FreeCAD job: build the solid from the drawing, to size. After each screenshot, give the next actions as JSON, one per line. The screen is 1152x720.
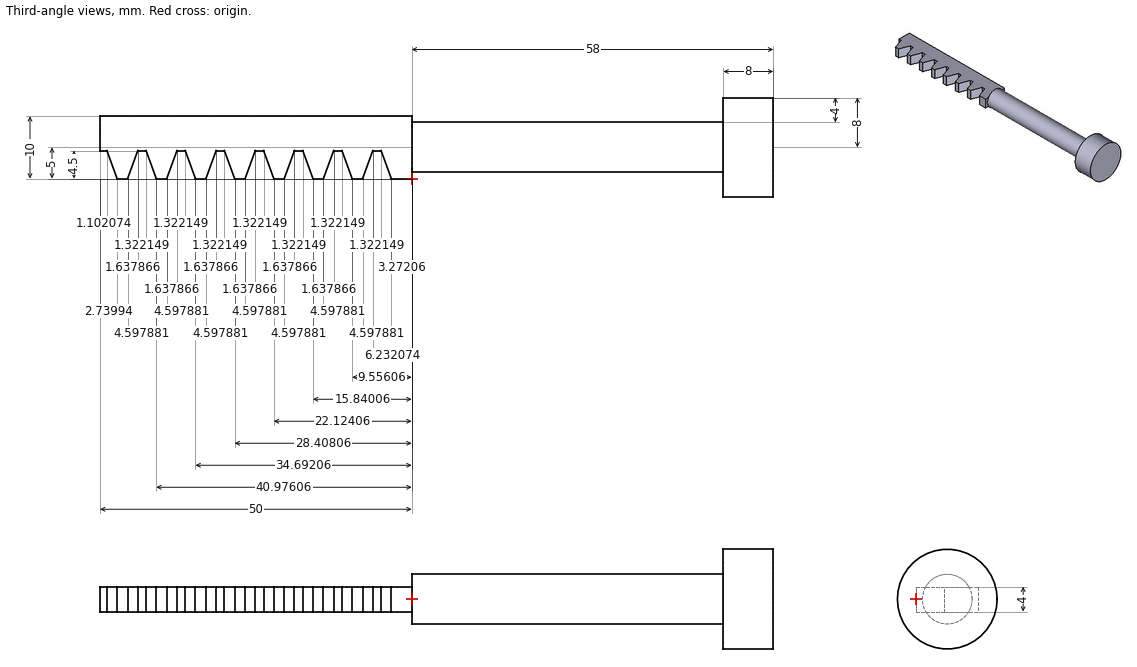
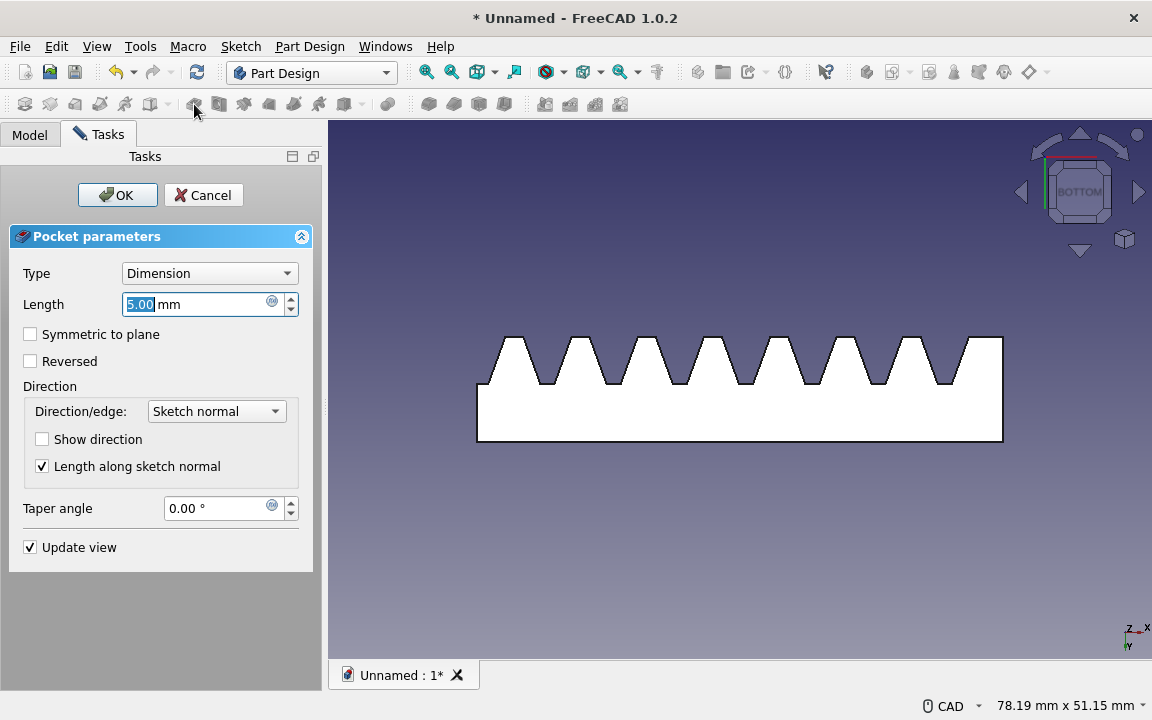
{"action": "left_click", "coordinate": [210, 274]}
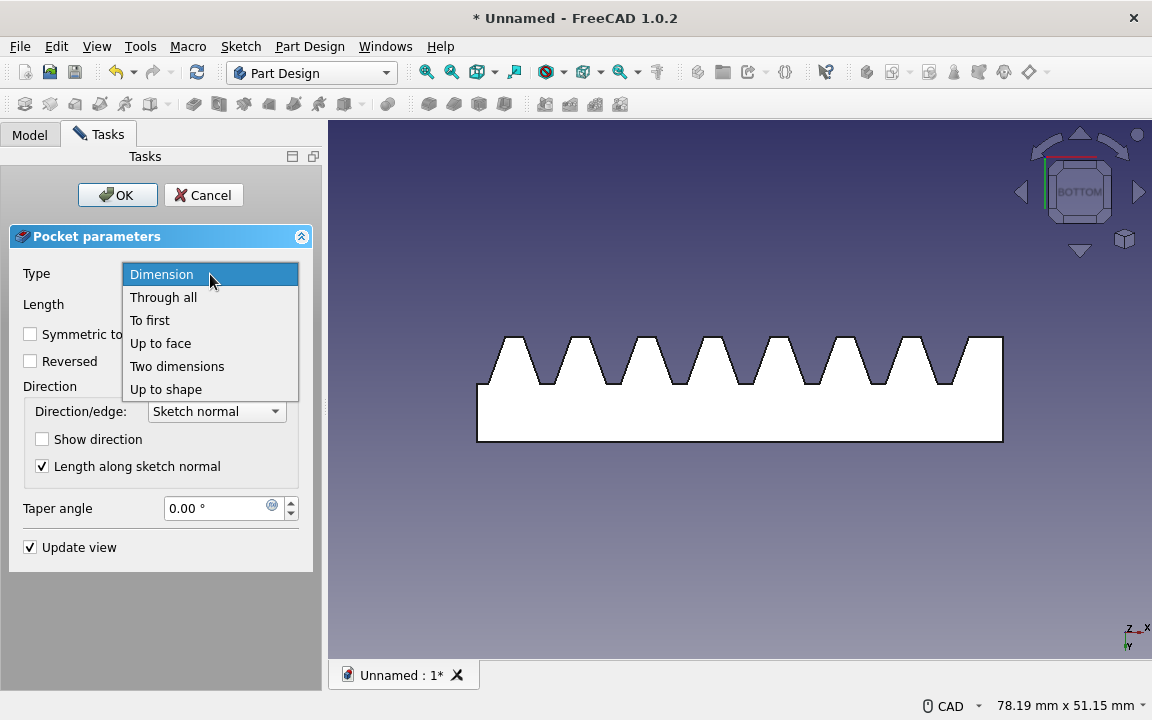
{"action": "left_click", "coordinate": [208, 298]}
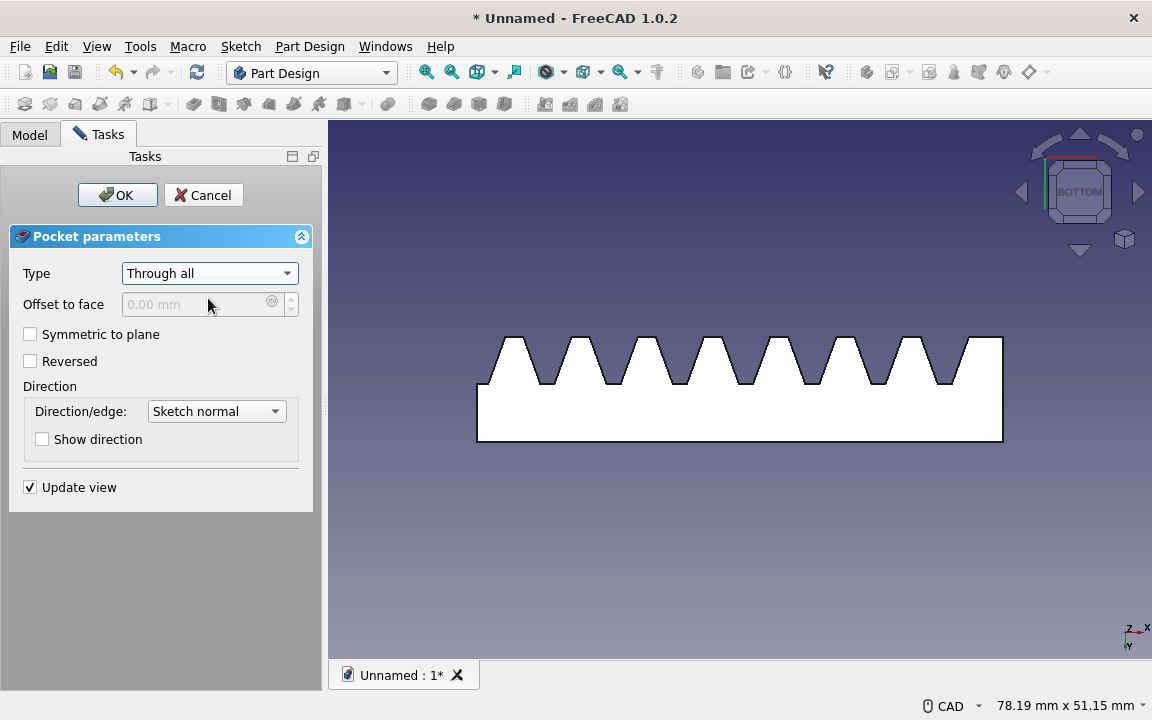
{"action": "left_click", "coordinate": [118, 195]}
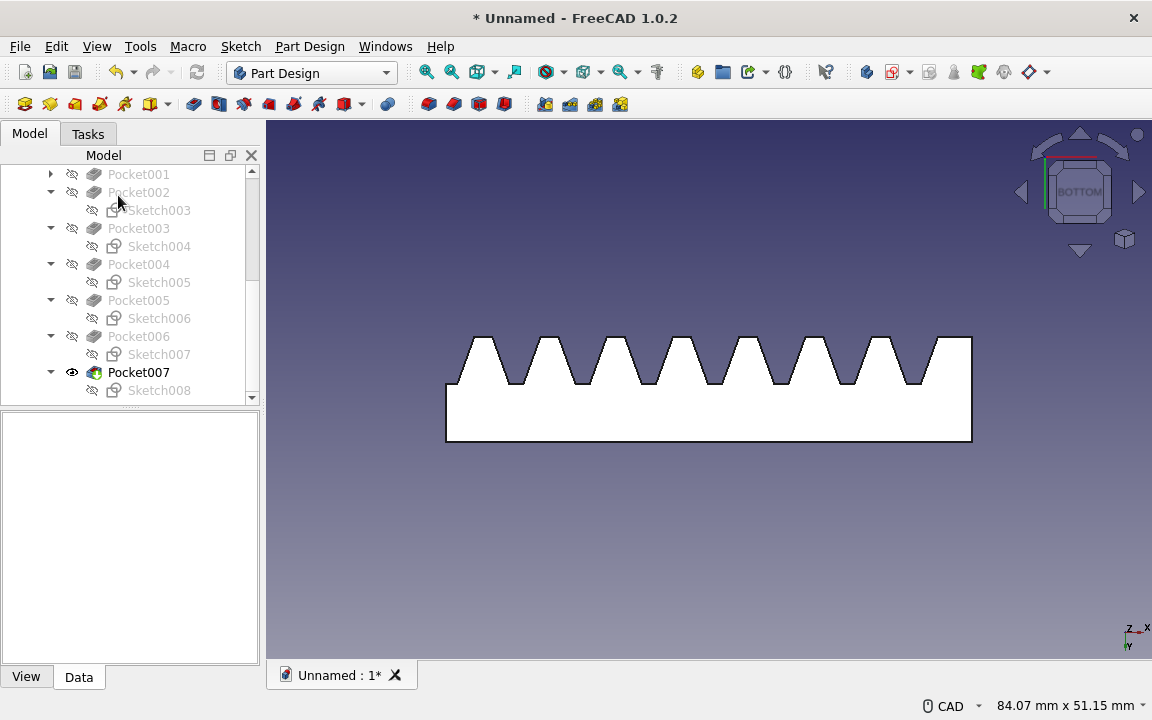
{"action": "left_click", "coordinate": [892, 72]}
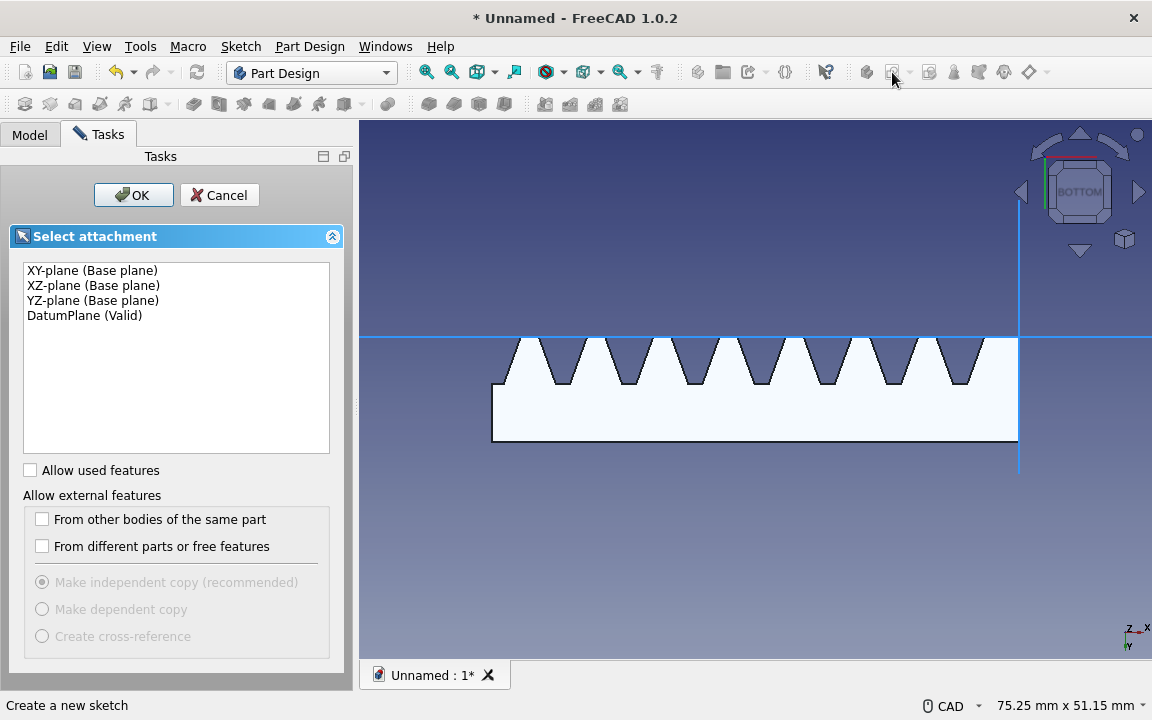
{"action": "left_click", "coordinate": [84, 270]}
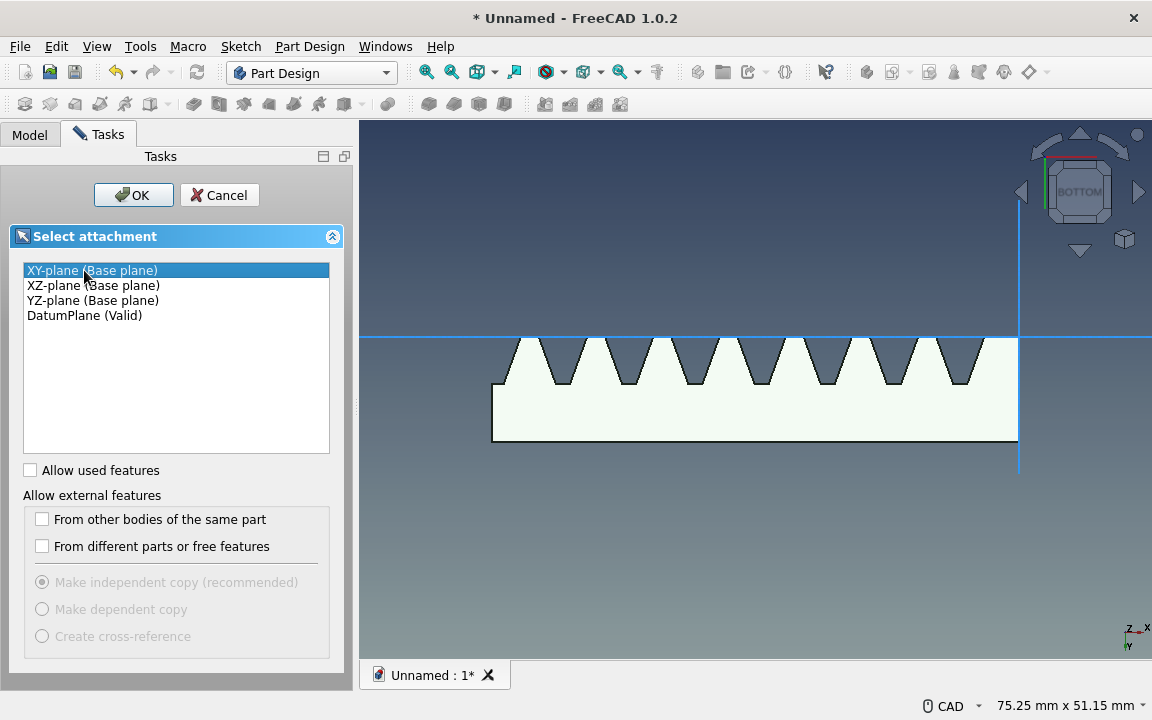
{"action": "left_click", "coordinate": [134, 195]}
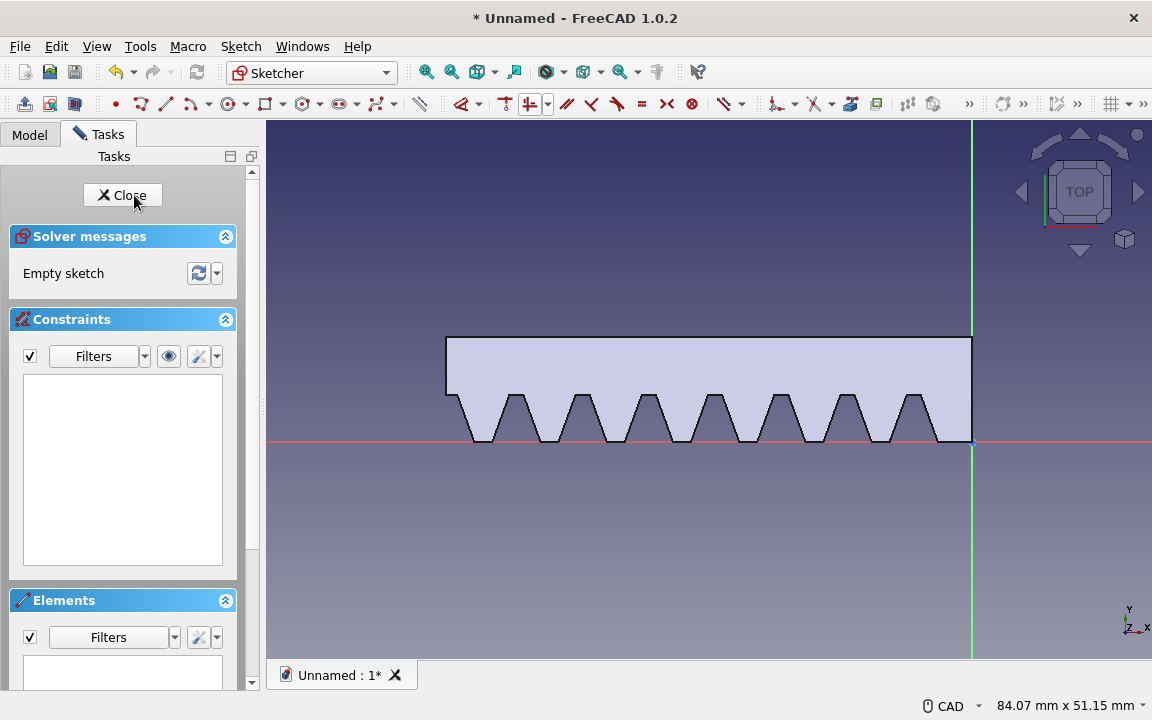
{"action": "left_click", "coordinate": [75, 104]}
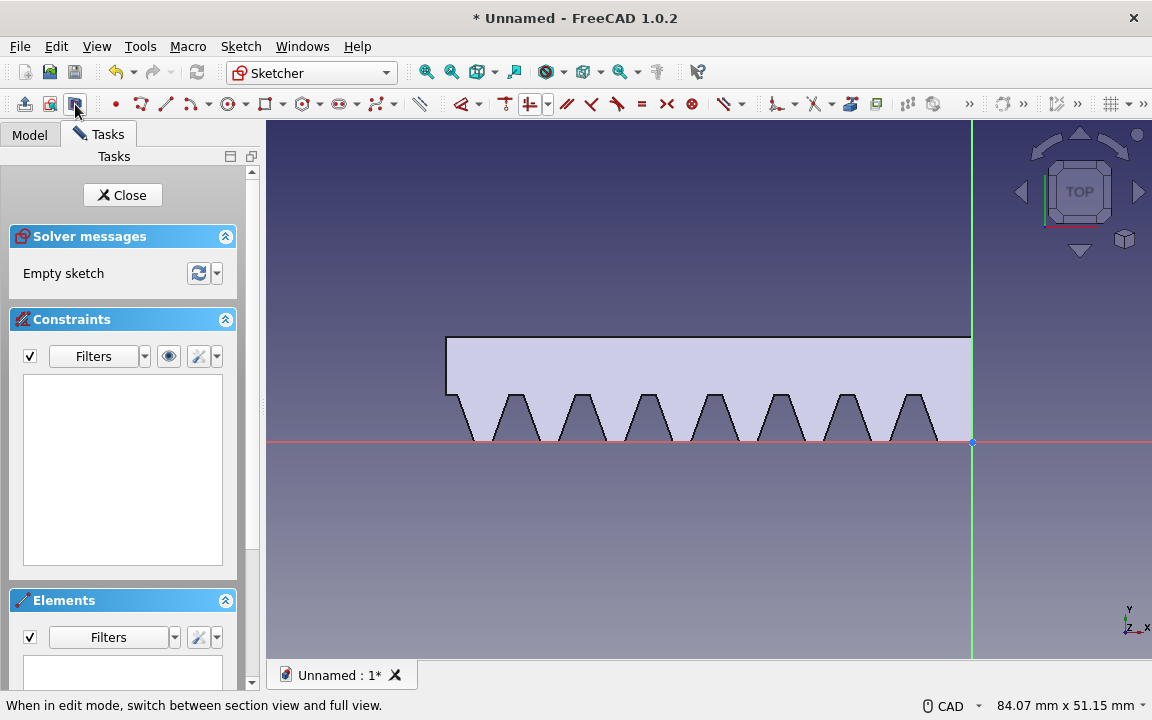
{"action": "scroll", "coordinate": [294, 399], "scroll_direction": "down", "scroll_amount": 5}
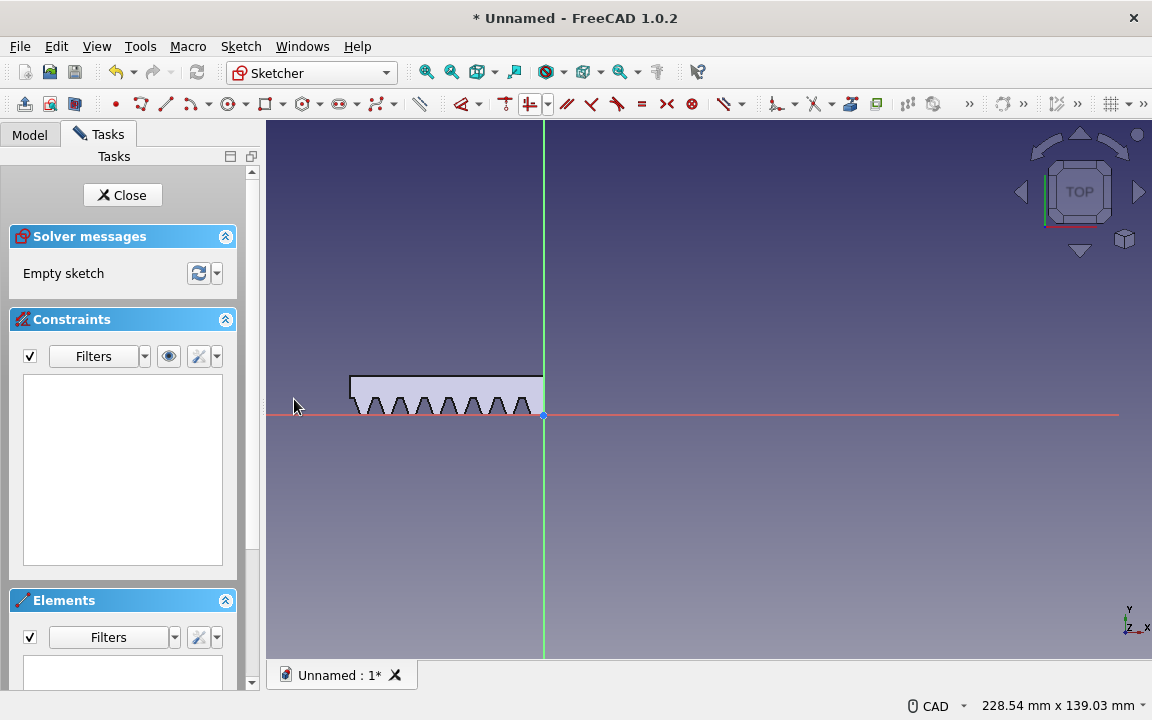
{"action": "scroll", "coordinate": [824, 391], "scroll_direction": "up", "scroll_amount": 2}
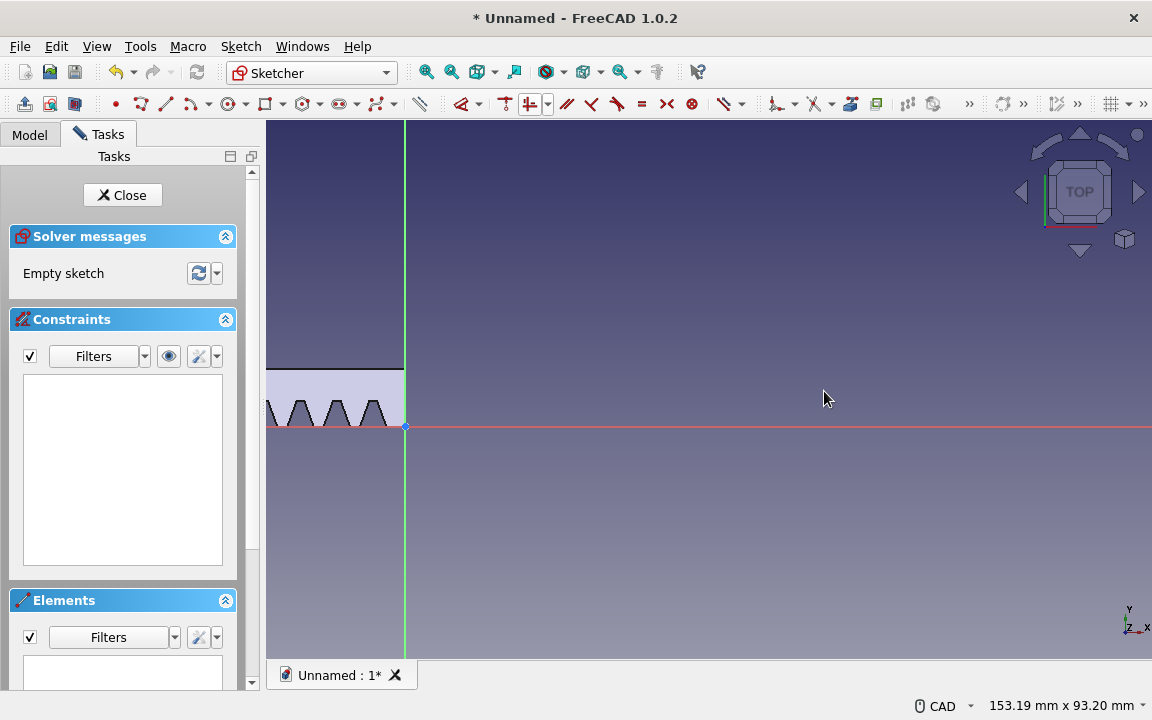
{"action": "left_click", "coordinate": [141, 104]}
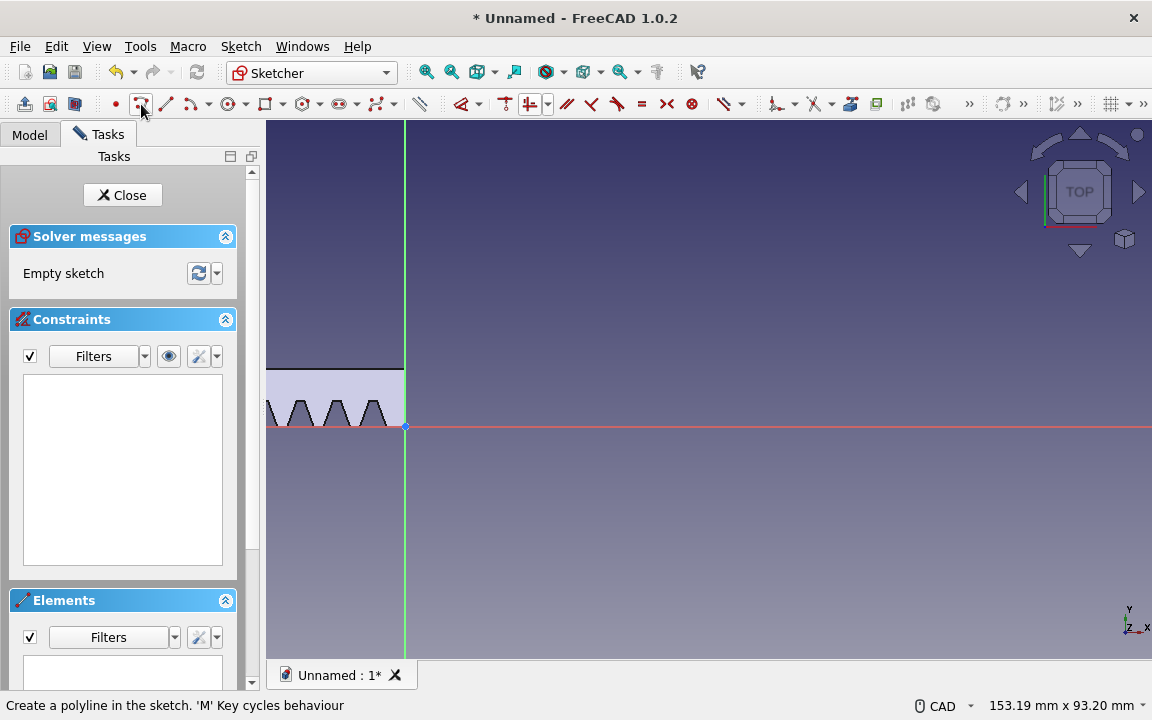
{"action": "left_click", "coordinate": [405, 398]}
{"action": "left_click", "coordinate": [741, 398]}
{"action": "left_click", "coordinate": [741, 352]}
{"action": "left_click", "coordinate": [695, 352]}
{"action": "left_click", "coordinate": [695, 375]}
{"action": "left_click", "coordinate": [414, 375]}
{"action": "left_click", "coordinate": [405, 399]}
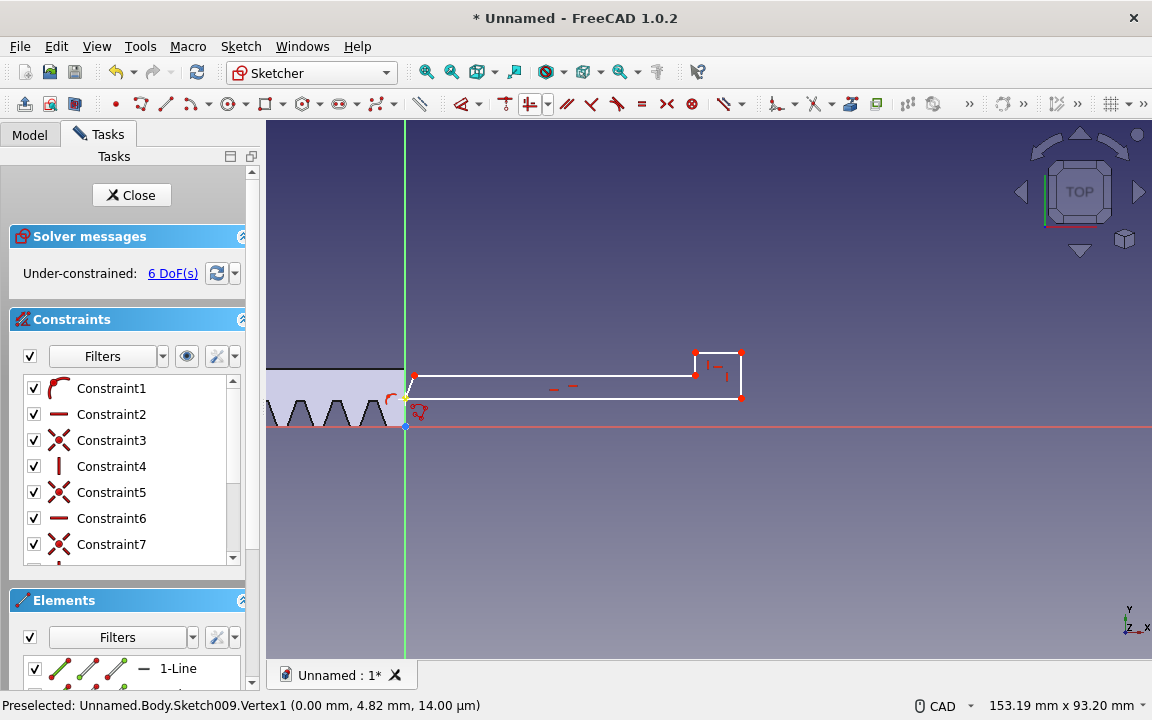
{"action": "left_click", "coordinate": [166, 104]}